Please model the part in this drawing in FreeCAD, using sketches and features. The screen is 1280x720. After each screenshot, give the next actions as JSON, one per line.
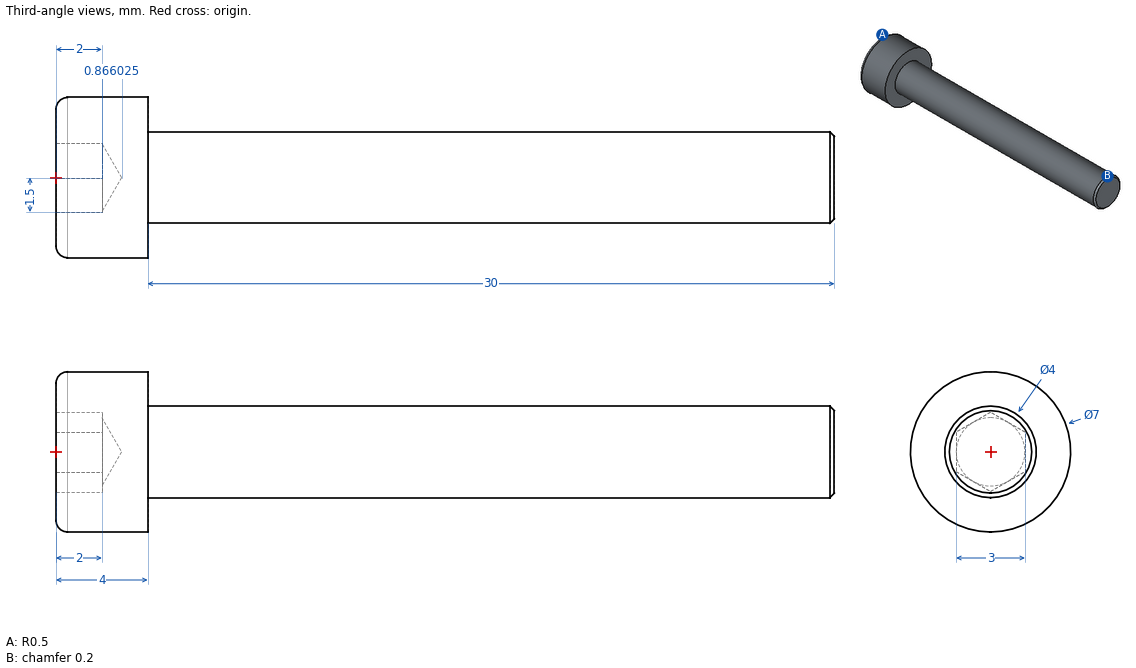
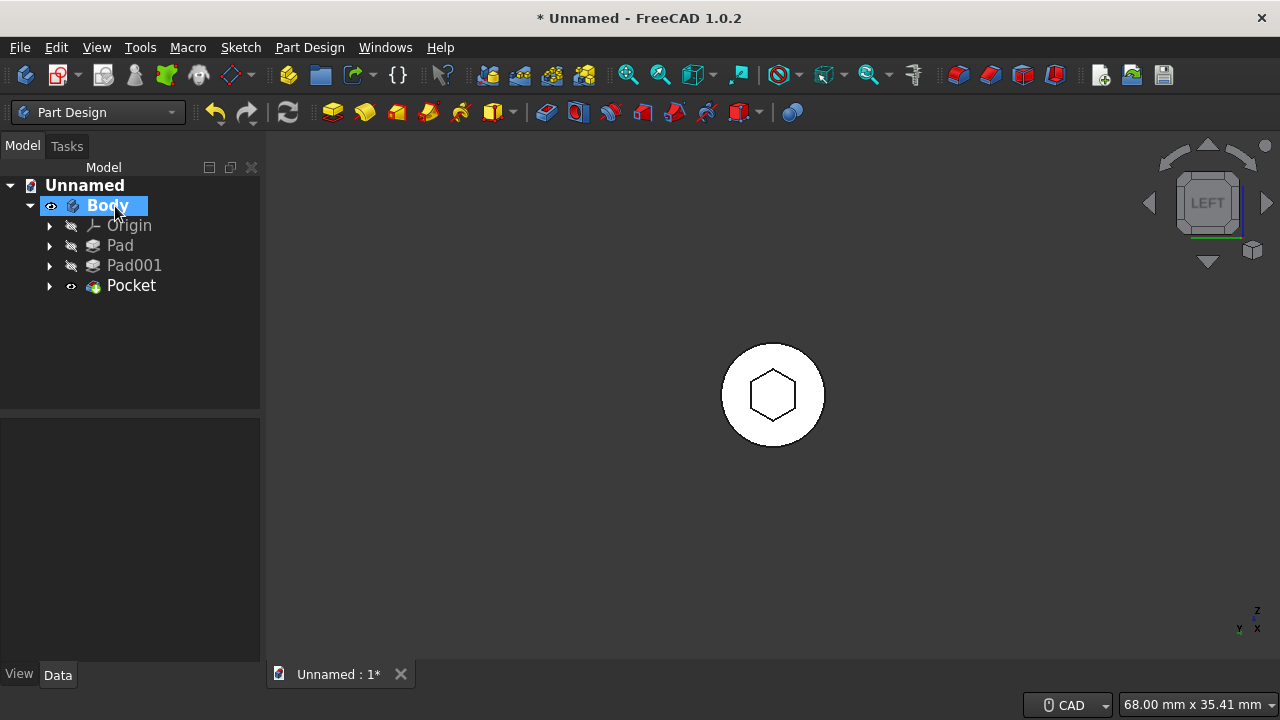
{"action": "left_click", "coordinate": [630, 76]}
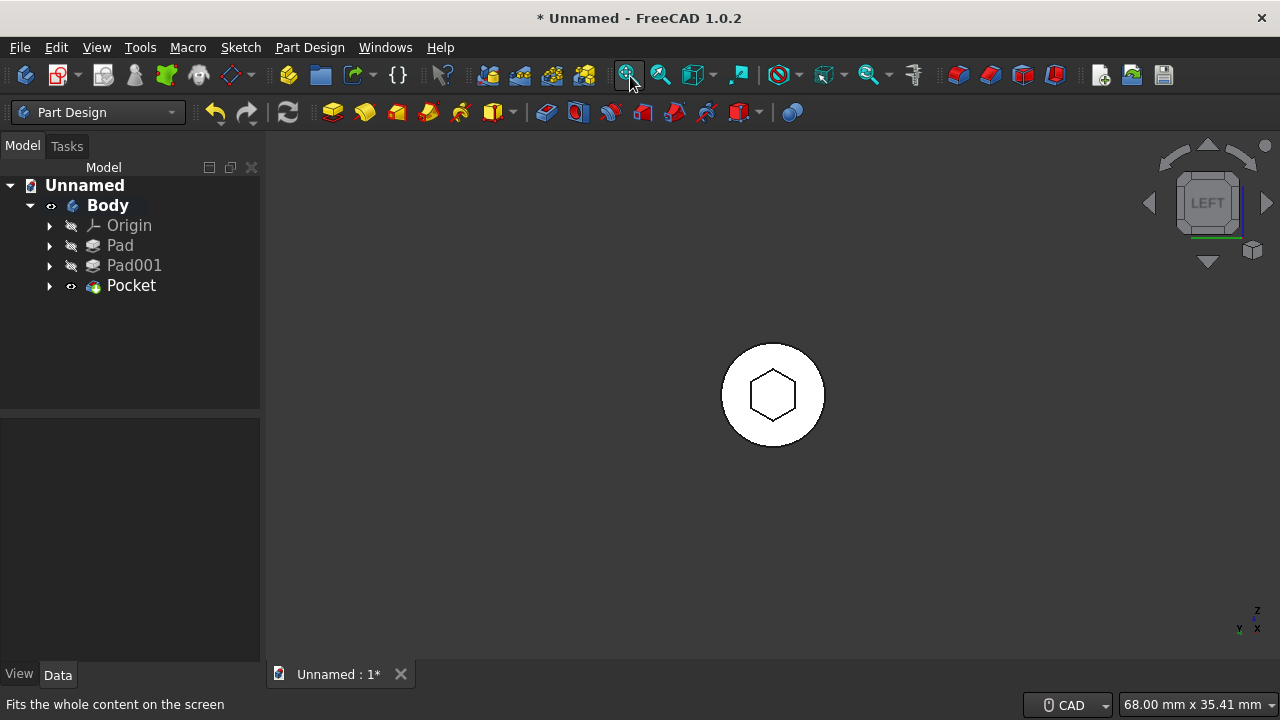
{"action": "left_click", "coordinate": [58, 76]}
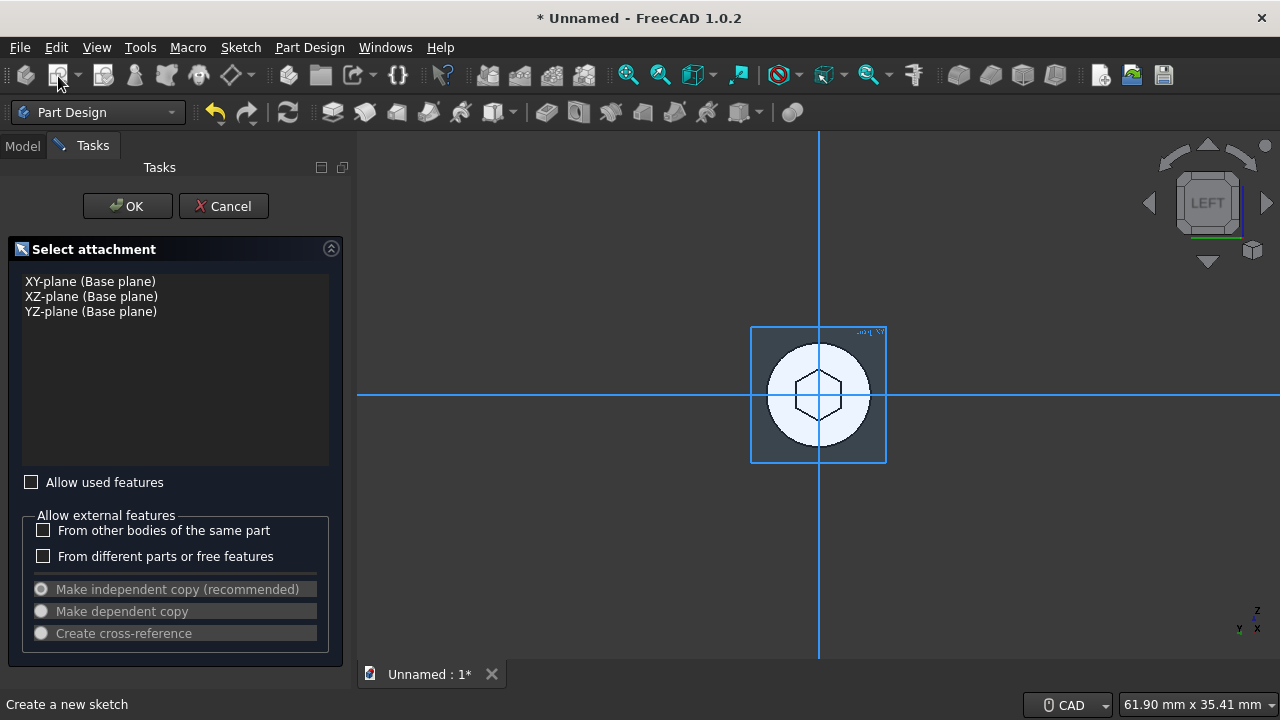
{"action": "left_click", "coordinate": [82, 282]}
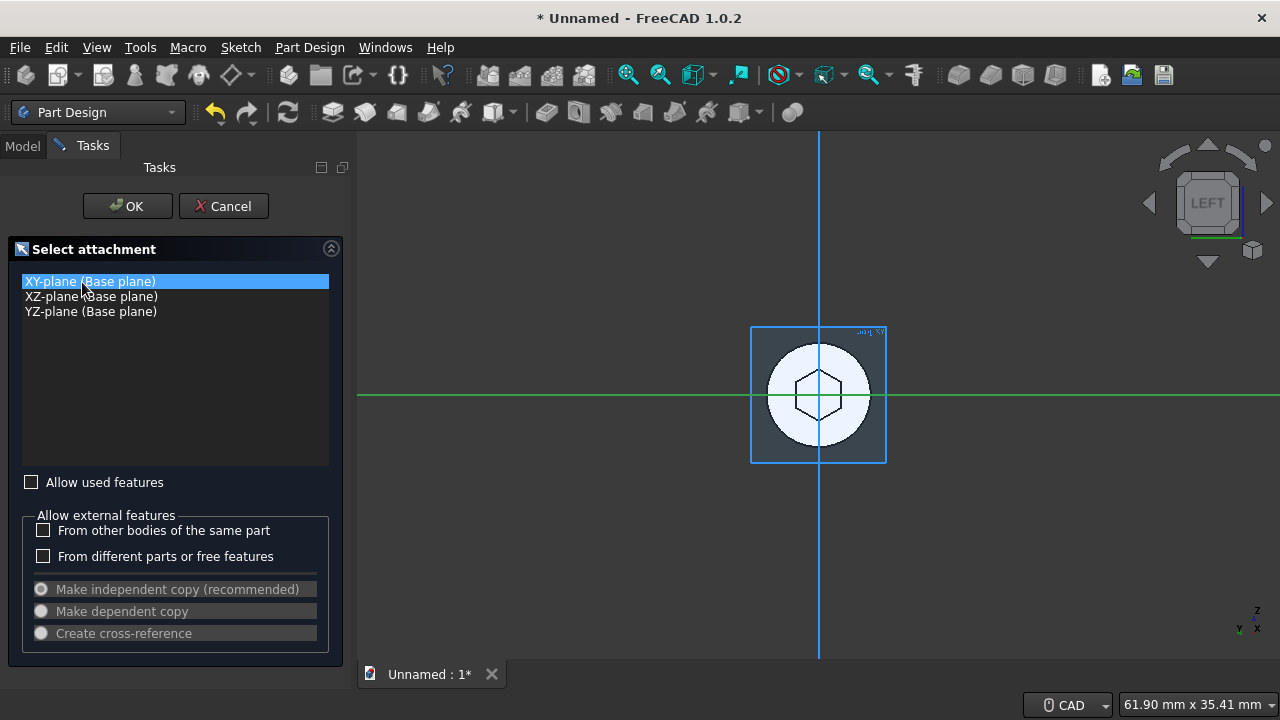
{"action": "left_click", "coordinate": [128, 206]}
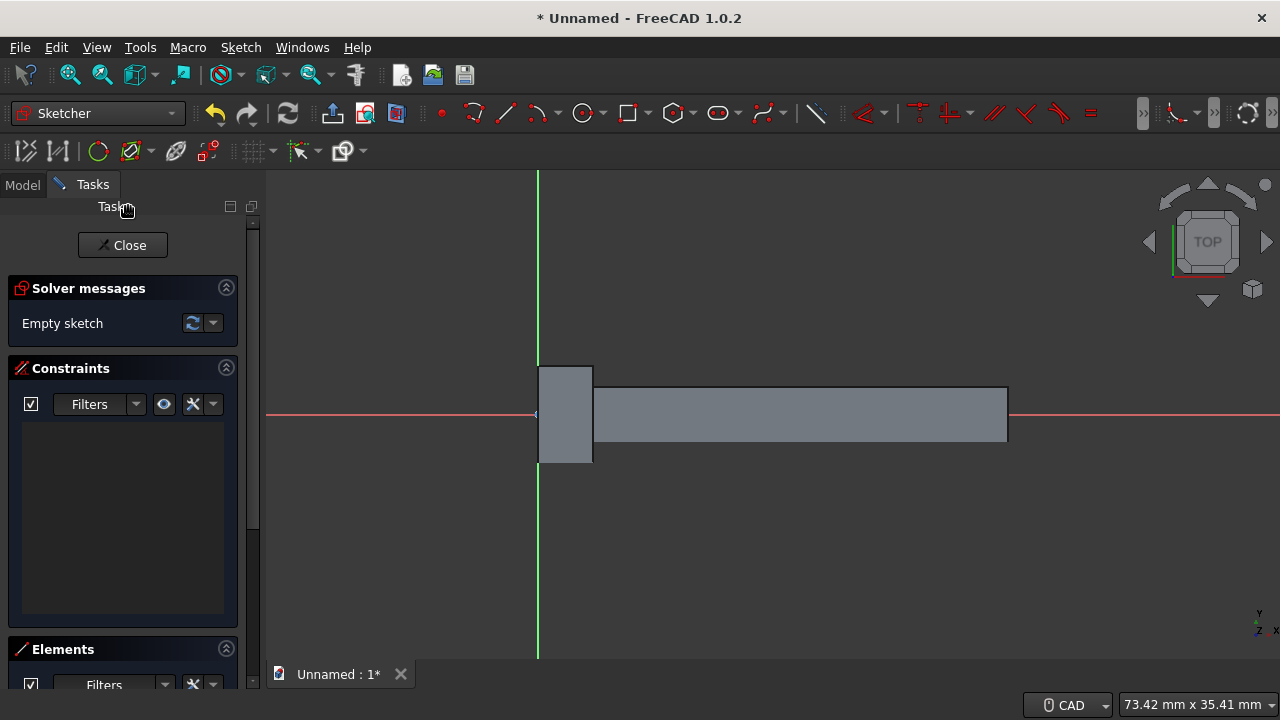
{"action": "left_click", "coordinate": [398, 114]}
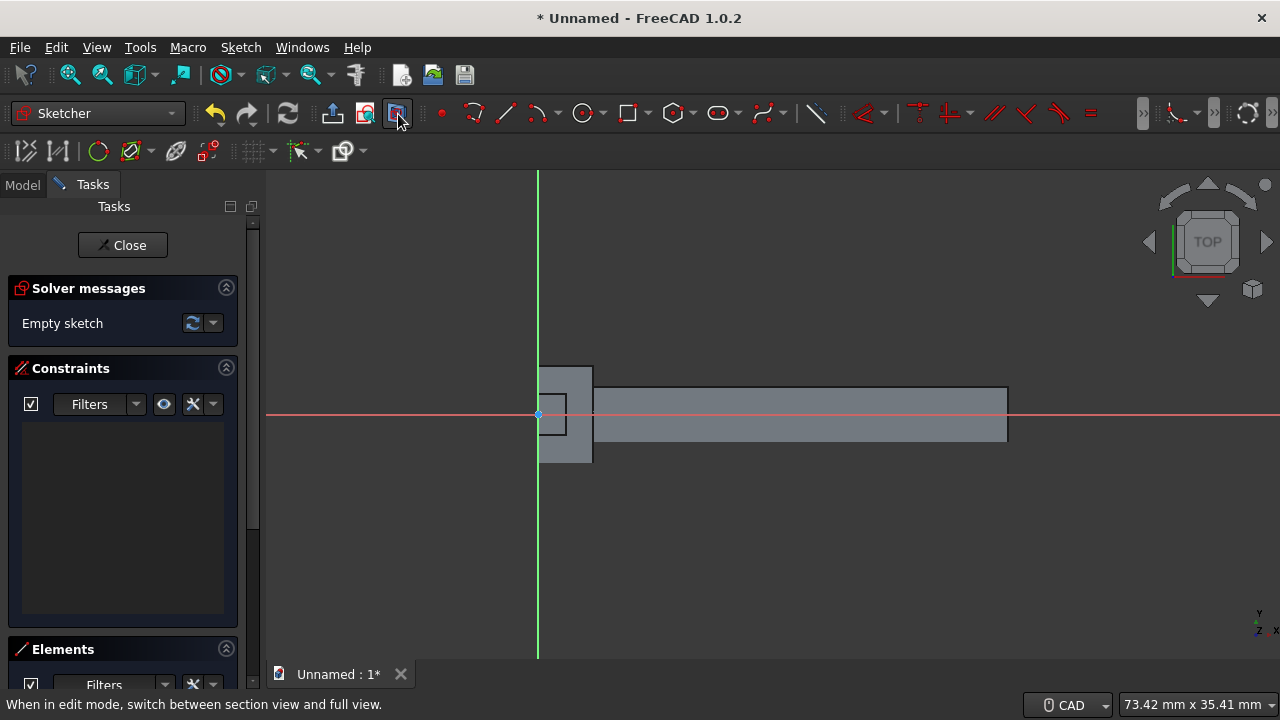
{"action": "scroll", "coordinate": [546, 426], "scroll_direction": "up", "scroll_amount": 13}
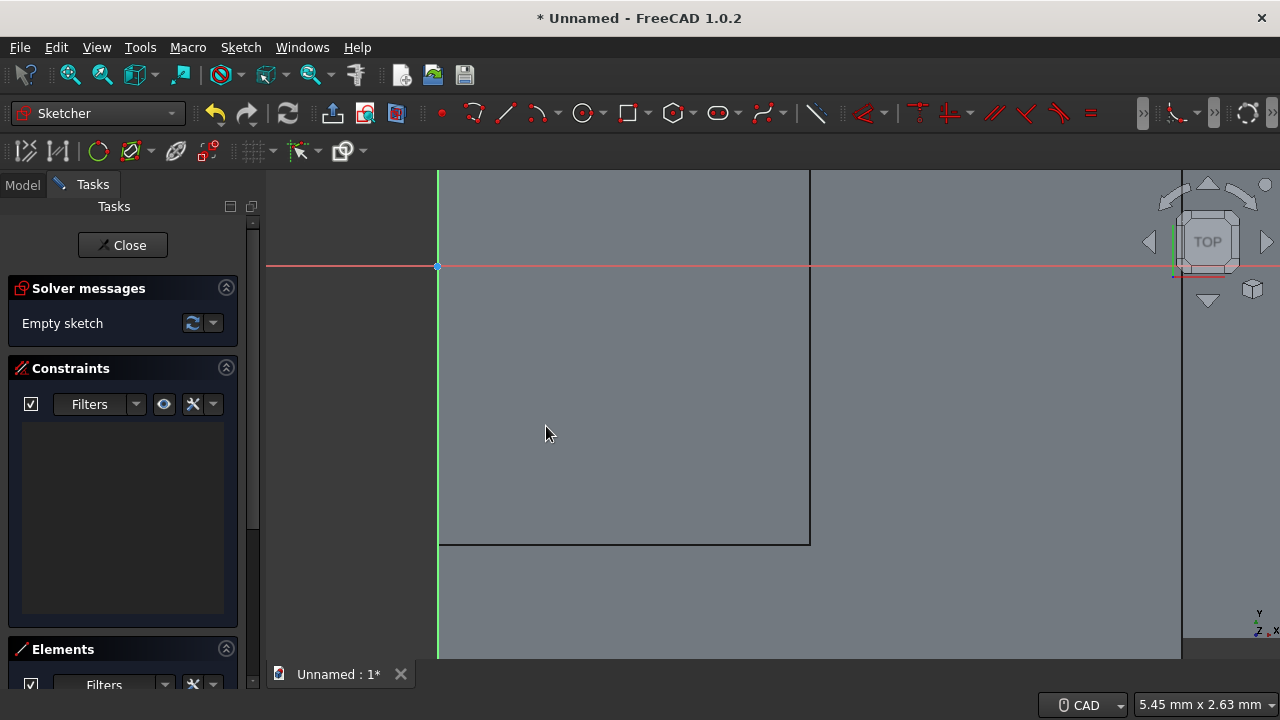
{"action": "left_click", "coordinate": [474, 114]}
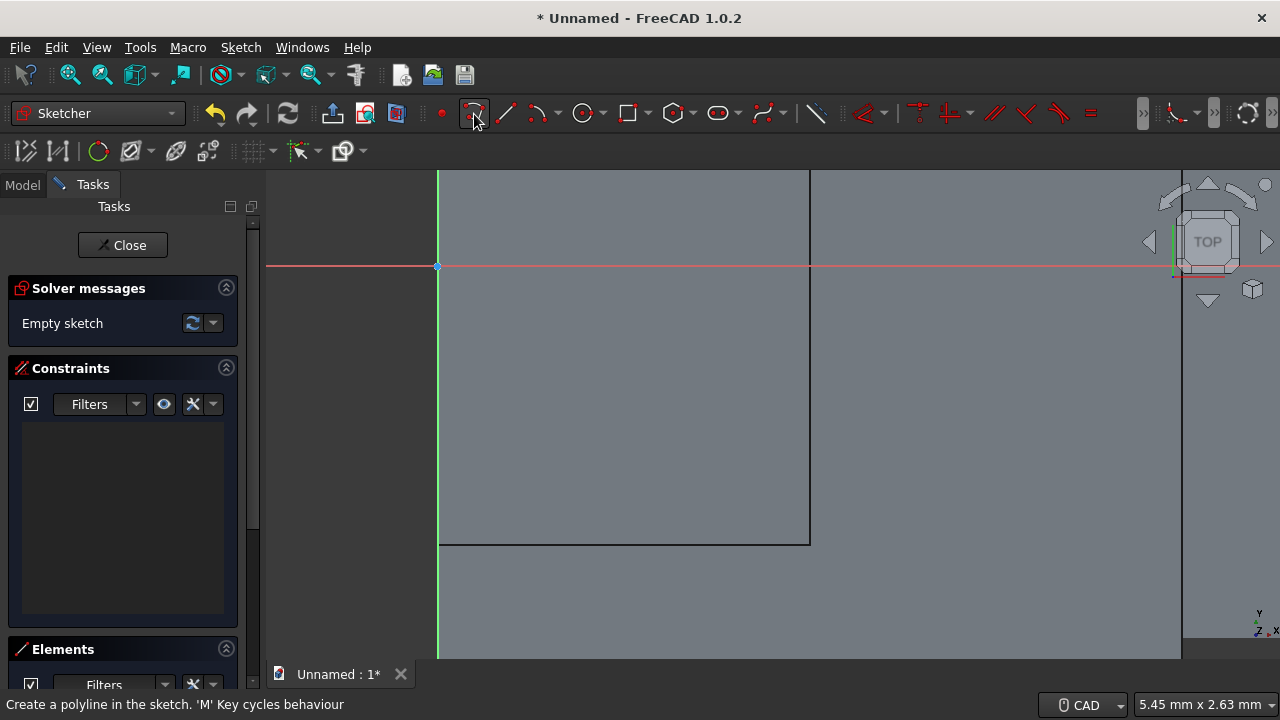
{"action": "left_click", "coordinate": [810, 266]}
{"action": "left_click", "coordinate": [810, 545]}
{"action": "left_click", "coordinate": [971, 275]}
{"action": "left_click", "coordinate": [810, 266]}
{"action": "key", "text": "Escape"}
{"action": "key", "text": "Escape"}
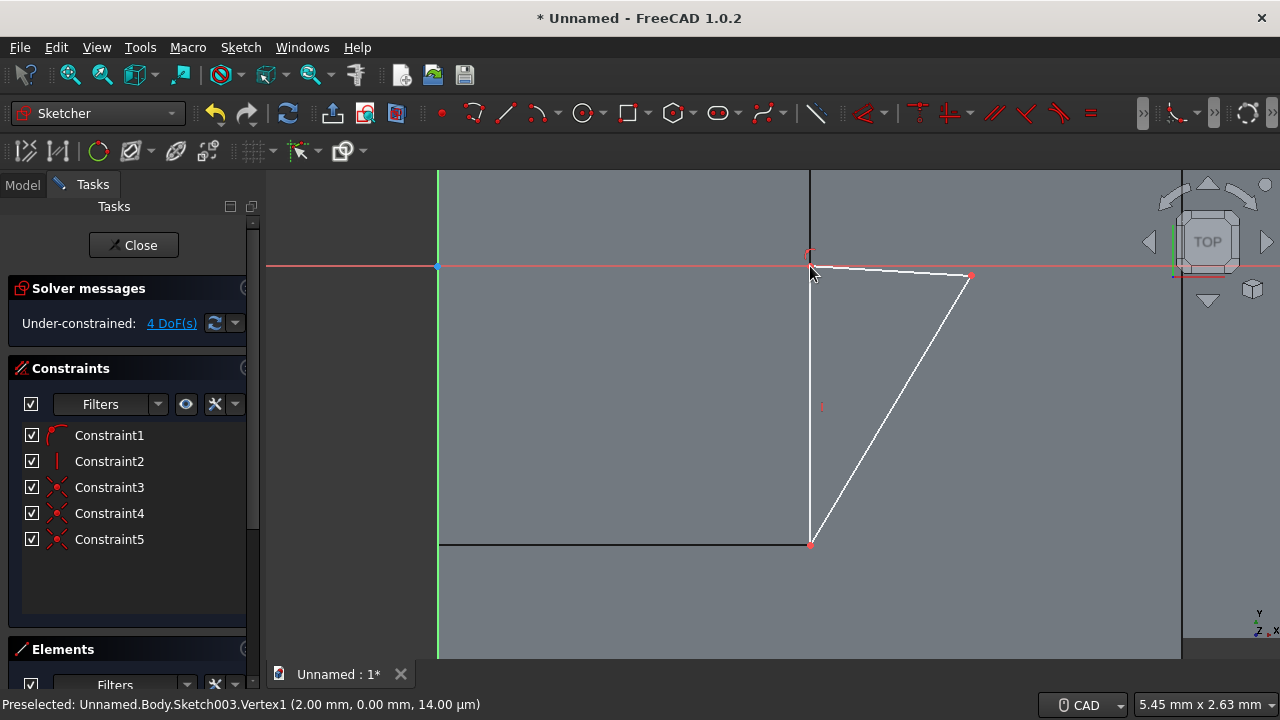
{"action": "left_click", "coordinate": [858, 269]}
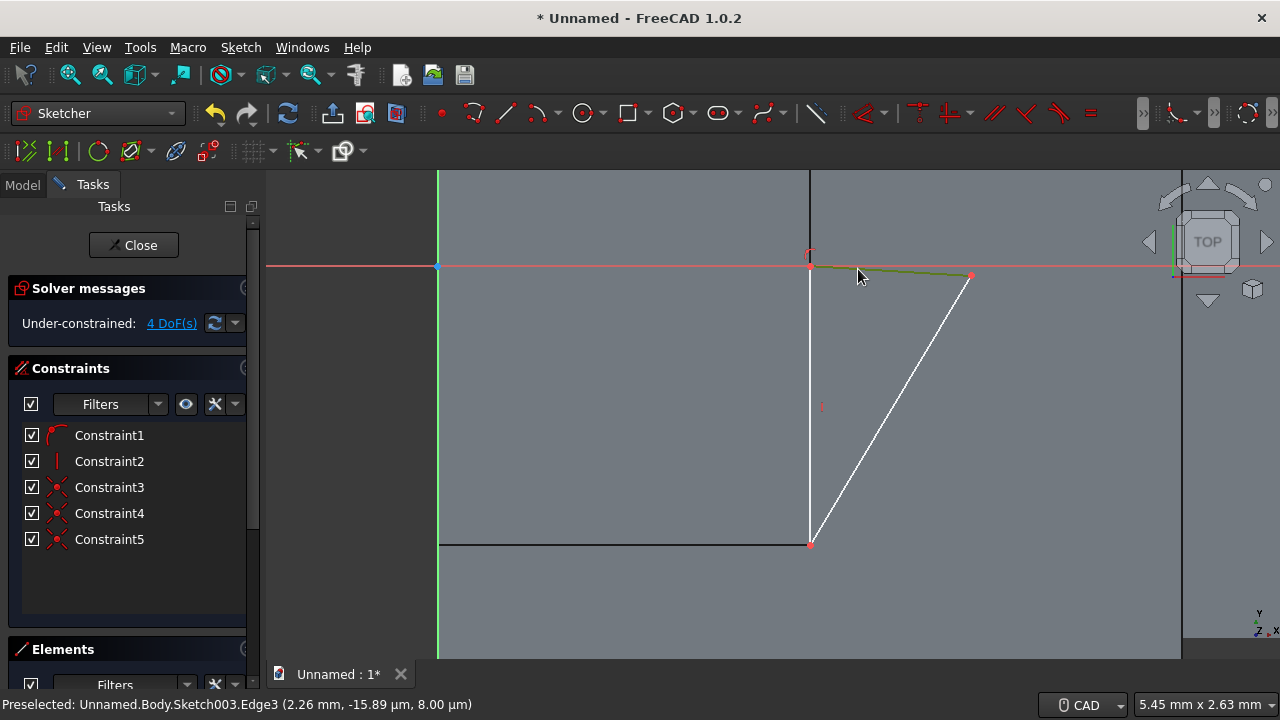
{"action": "key", "text": "h"}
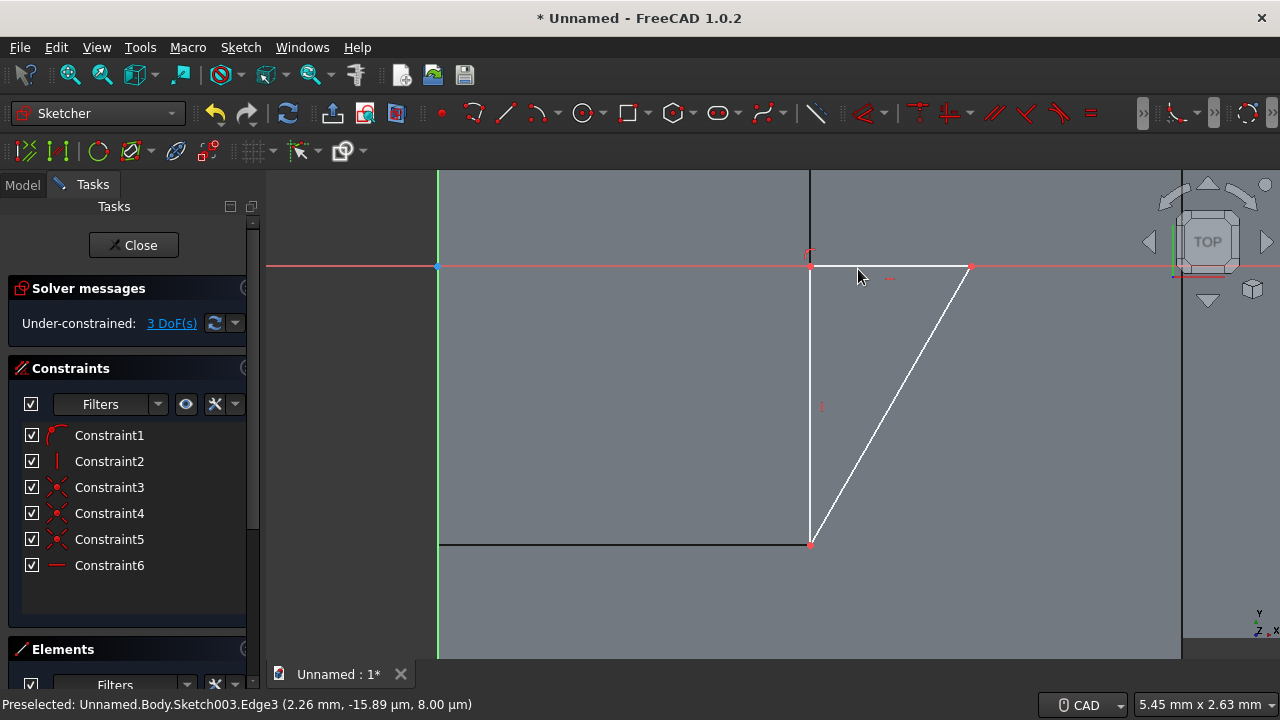
{"action": "left_click", "coordinate": [864, 114]}